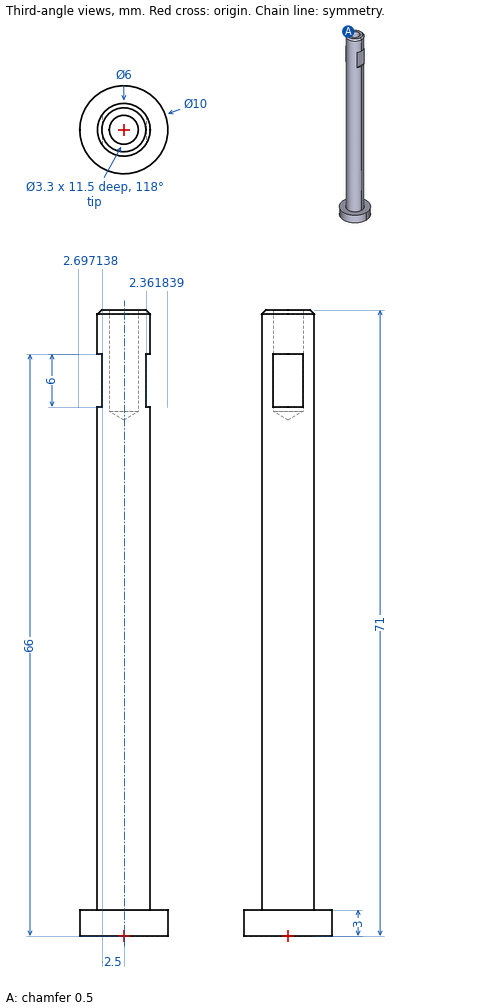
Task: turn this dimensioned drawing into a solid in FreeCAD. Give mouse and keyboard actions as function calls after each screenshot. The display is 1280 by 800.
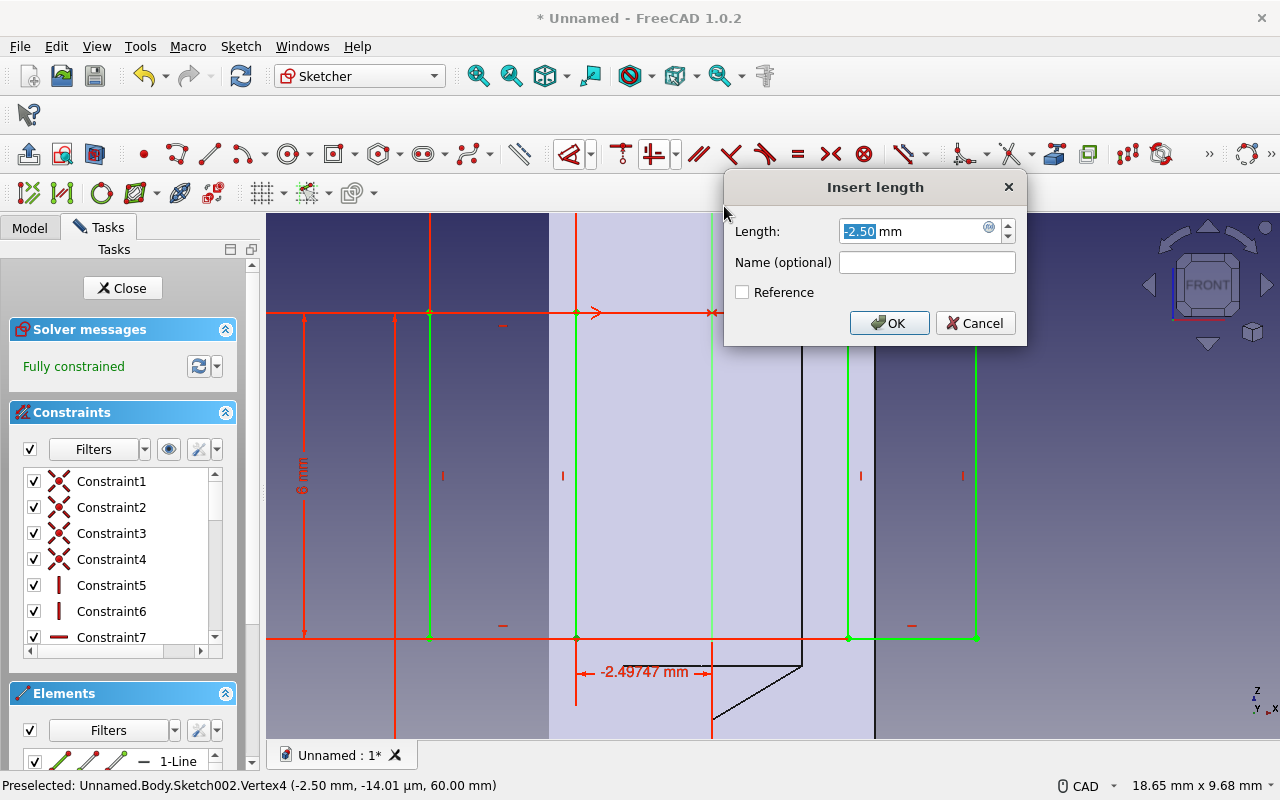
text(-2.5)
key(Return)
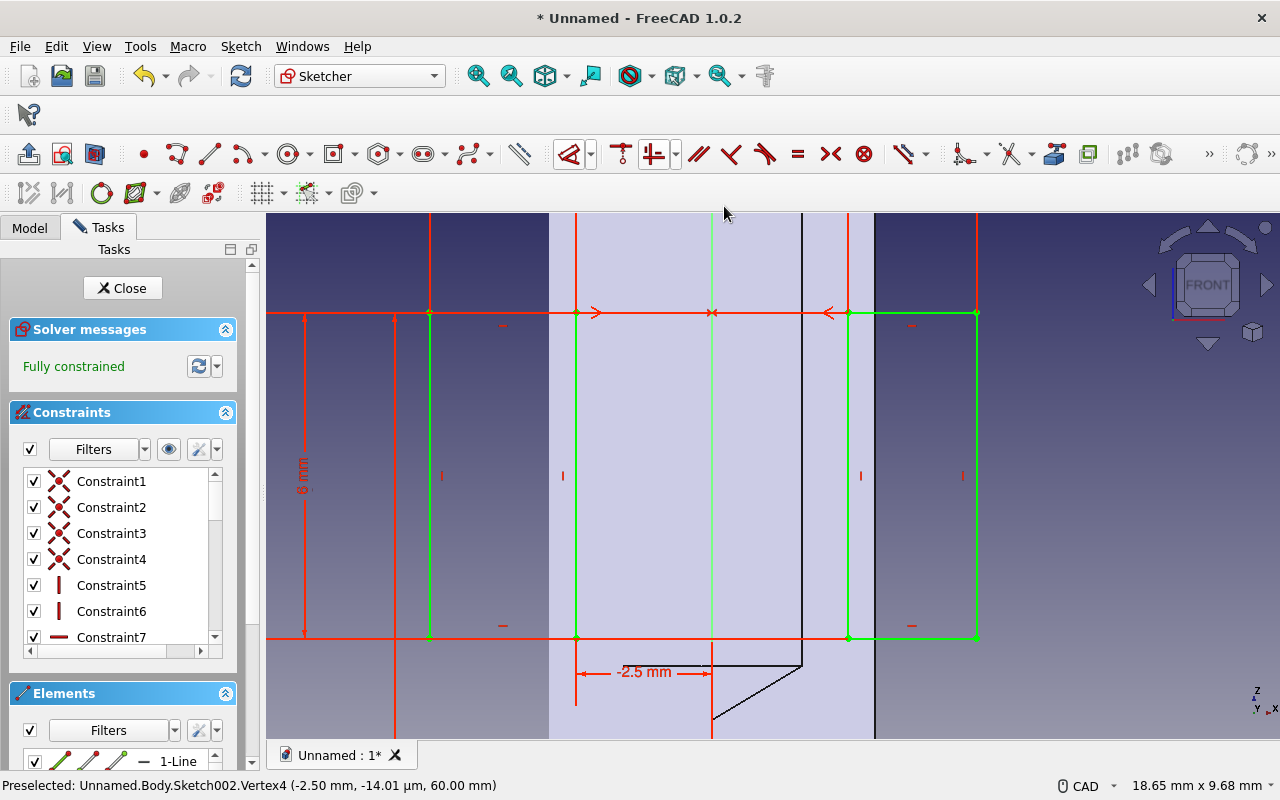
click(123, 288)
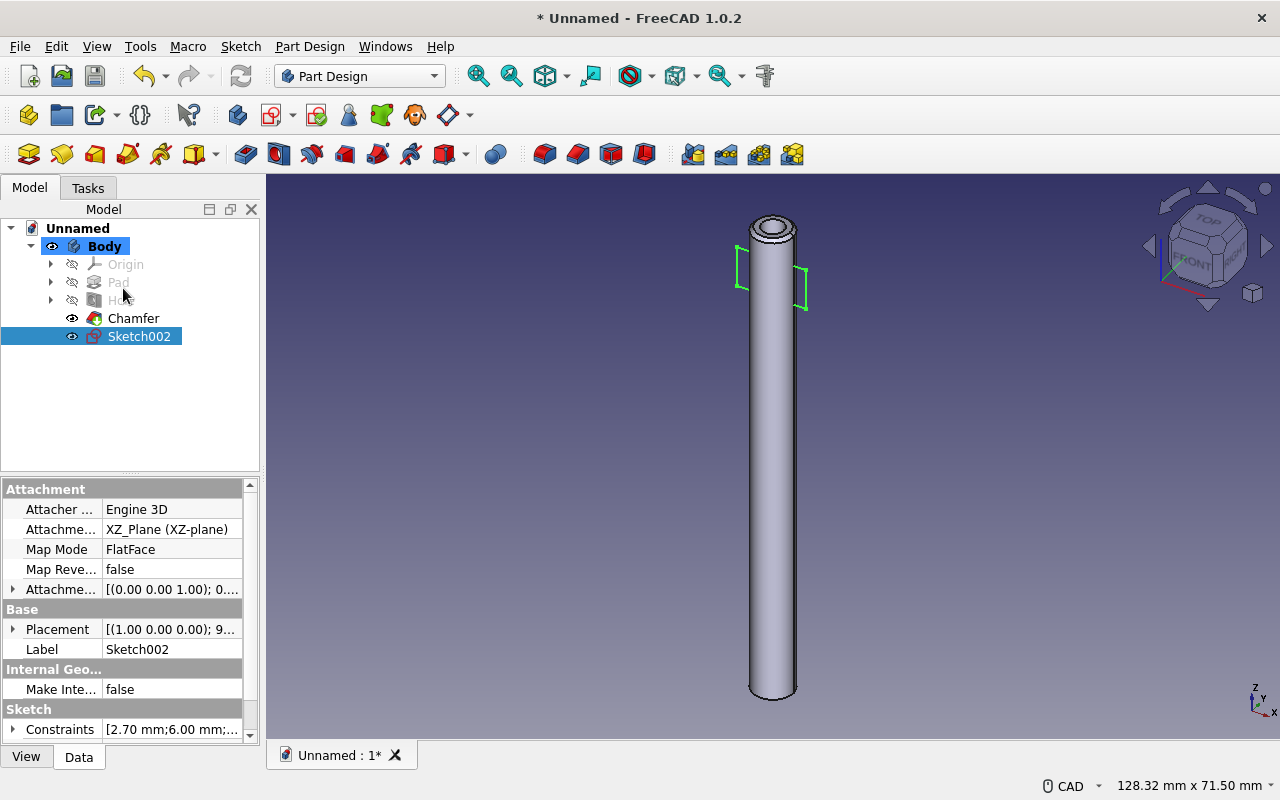
click(246, 154)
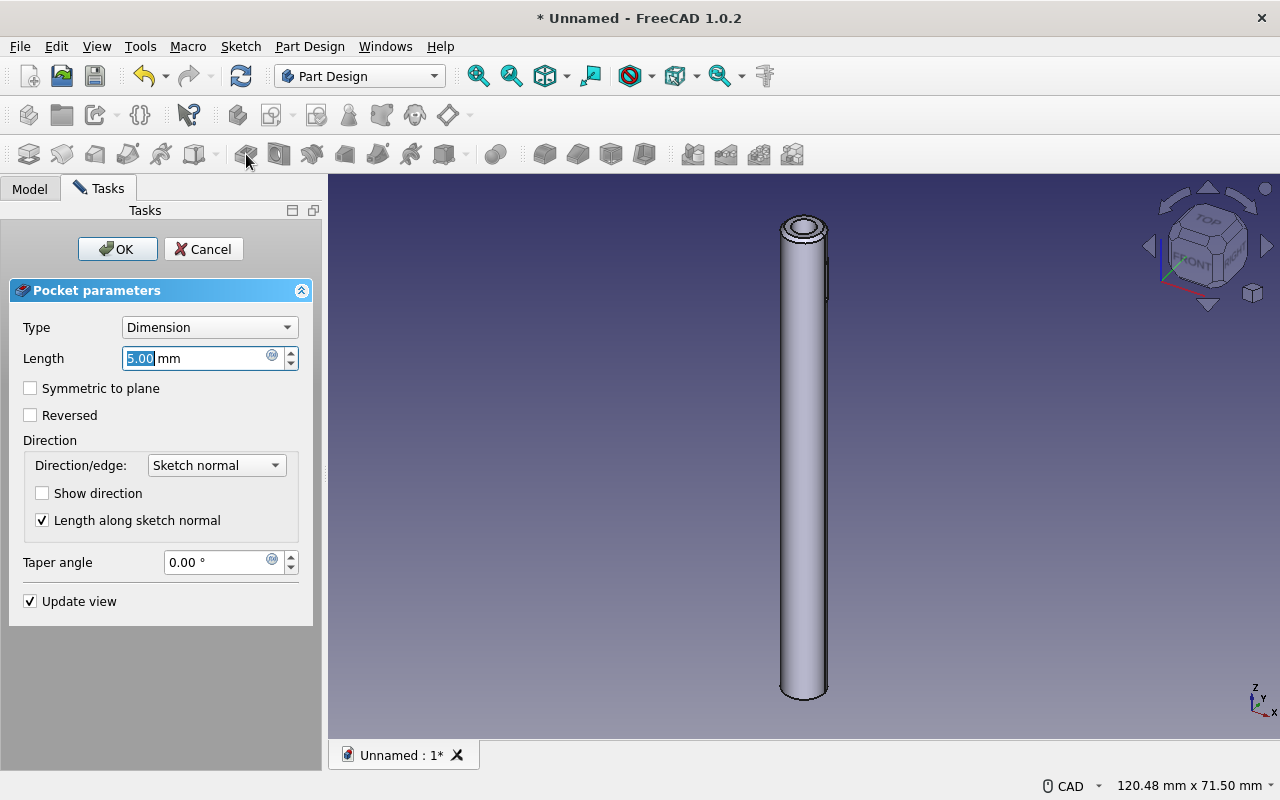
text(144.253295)
key(Tab)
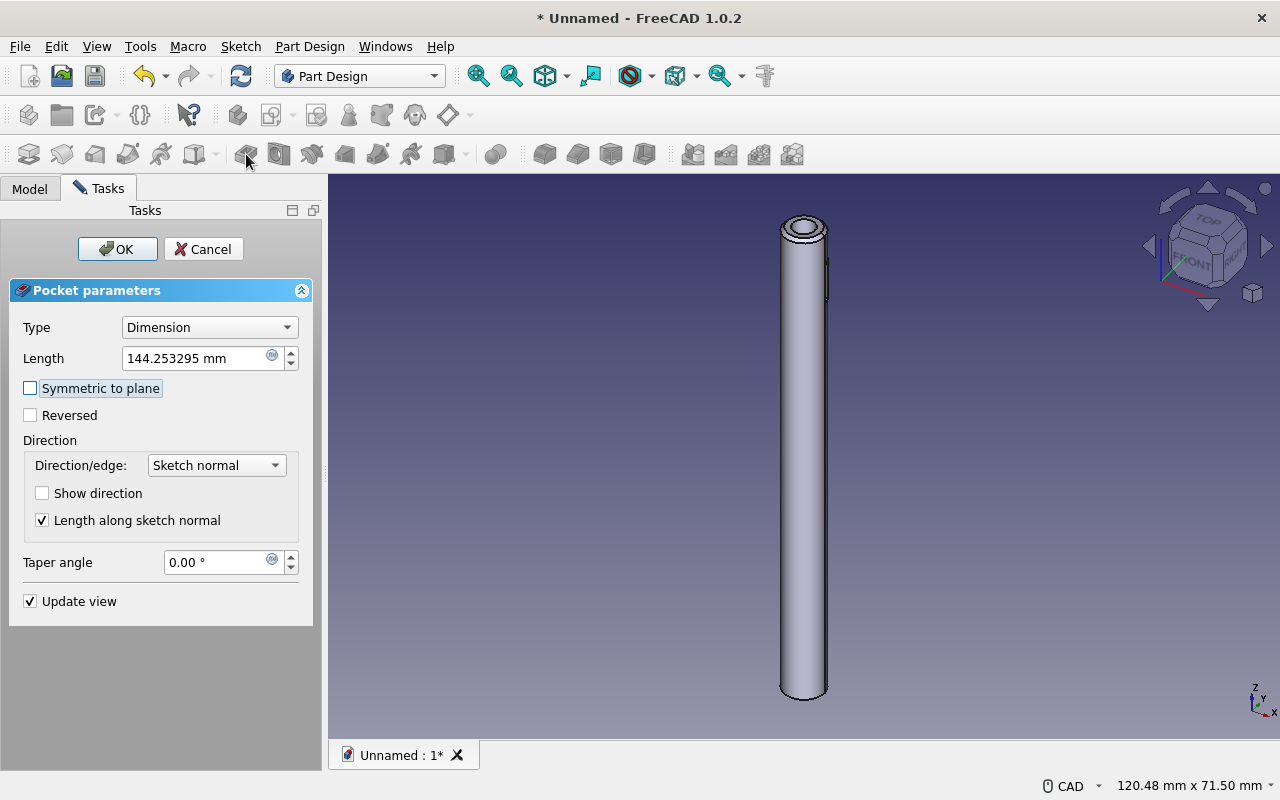
click(31, 388)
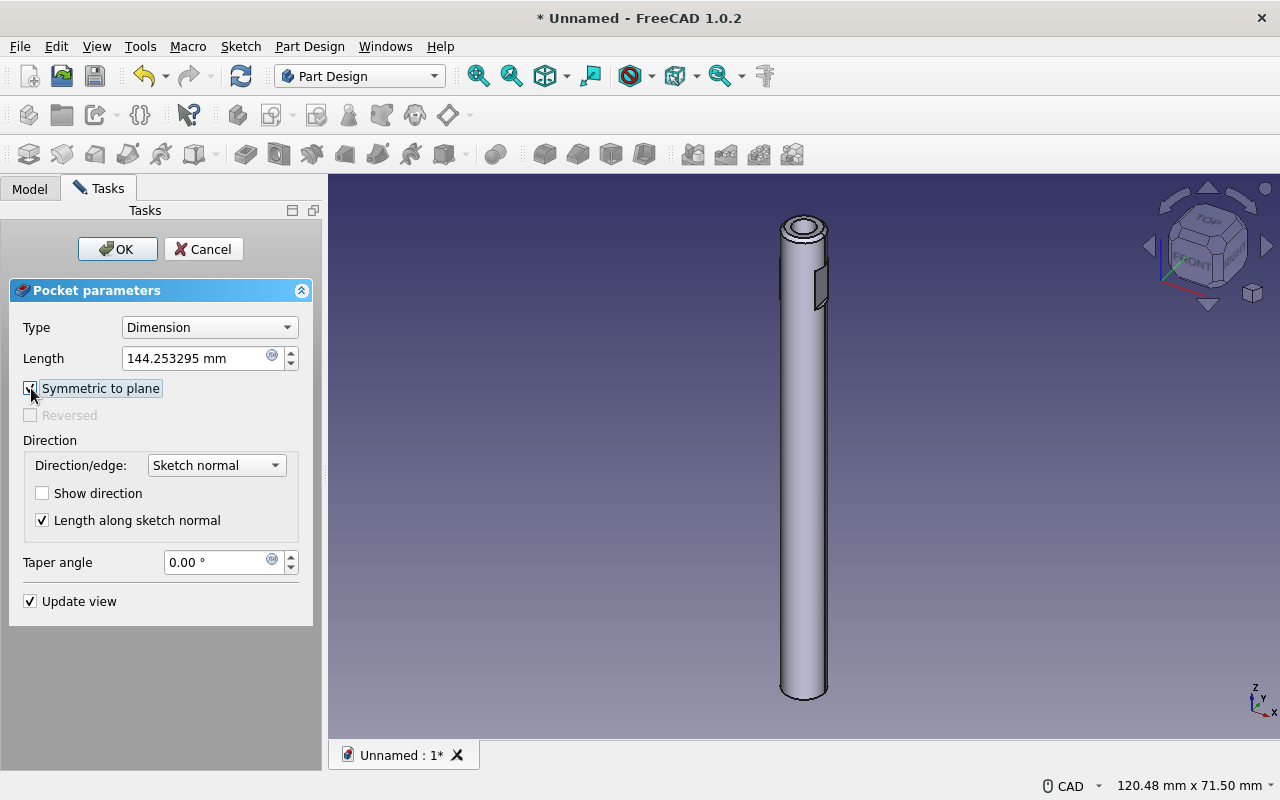
click(118, 249)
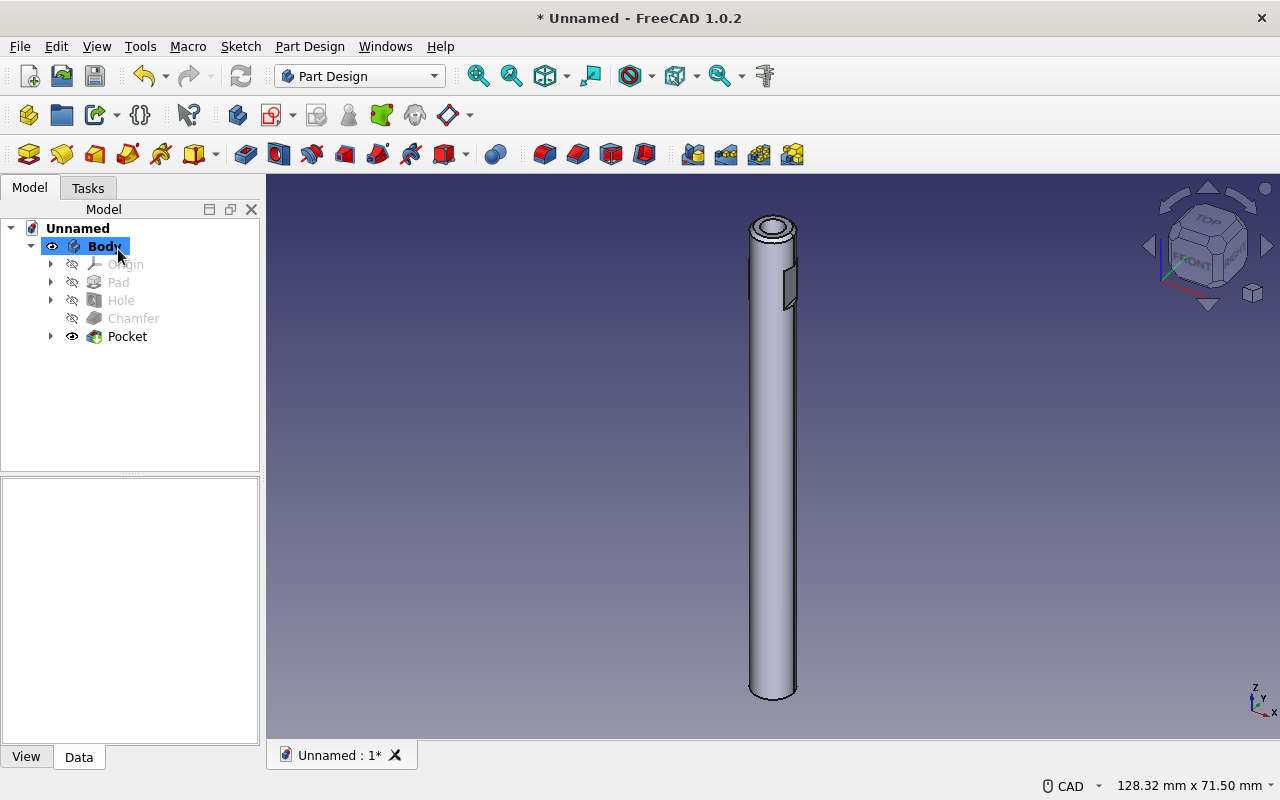
click(270, 116)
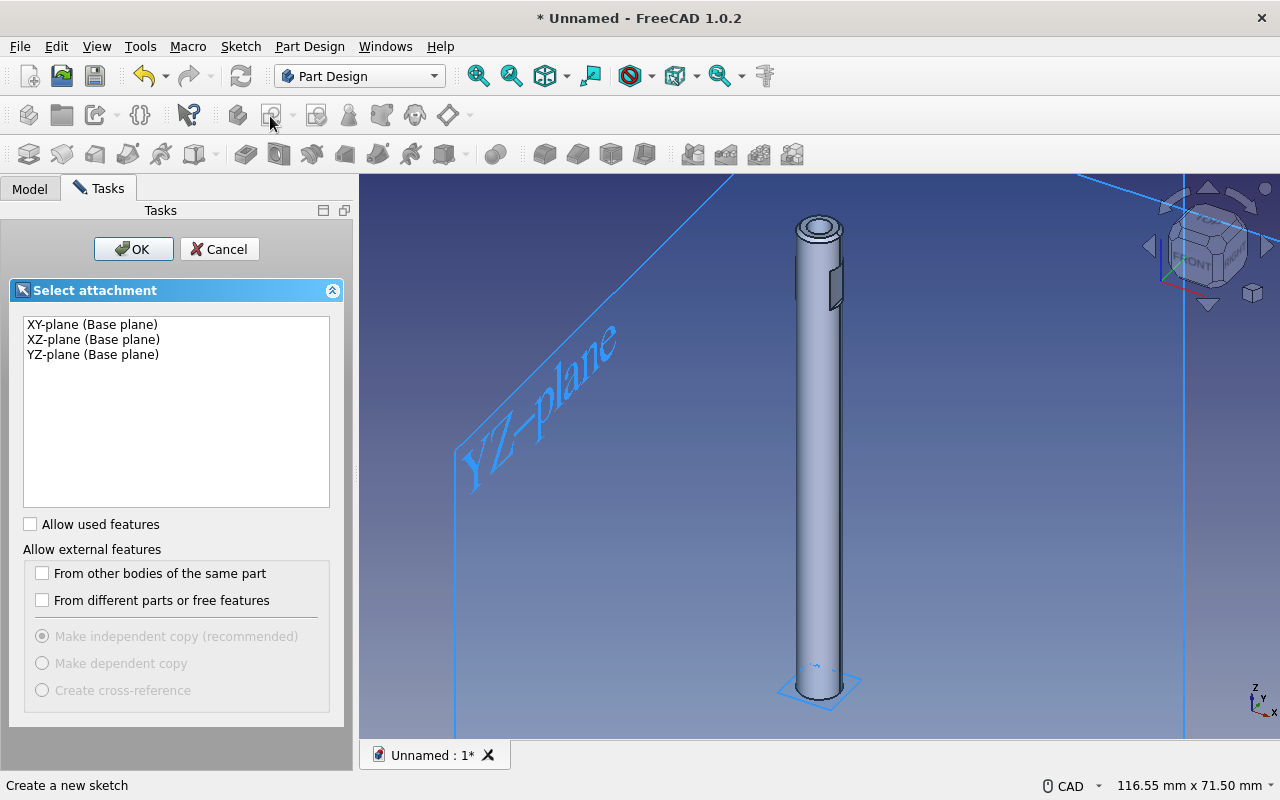
click(84, 324)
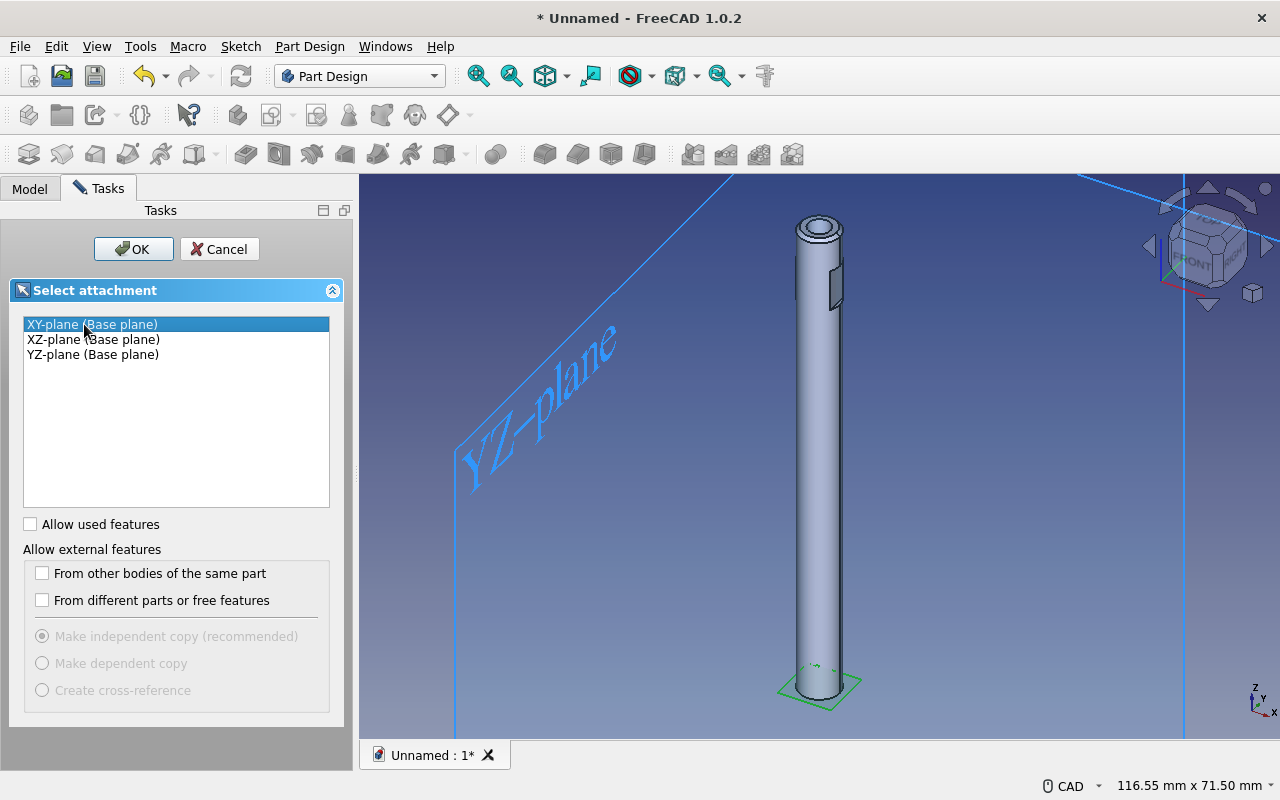
click(134, 249)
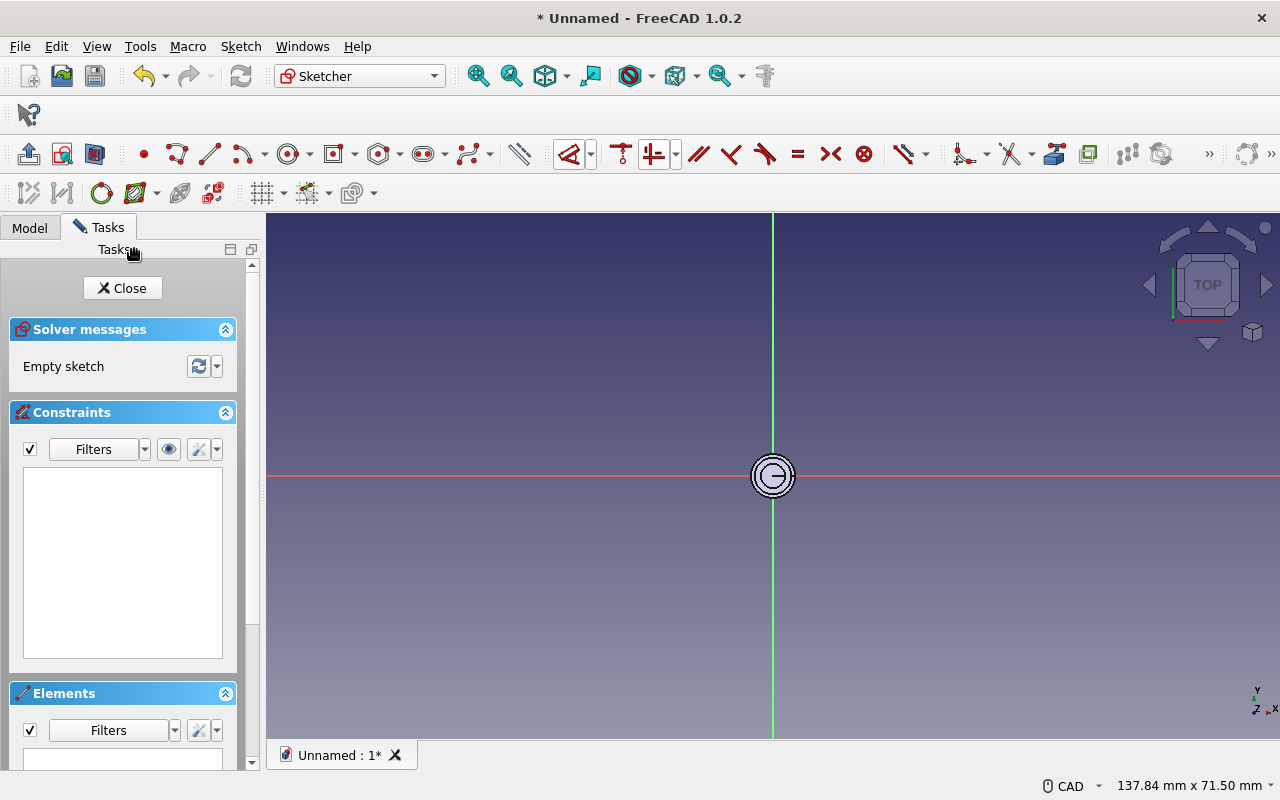
key(q)
key(s)